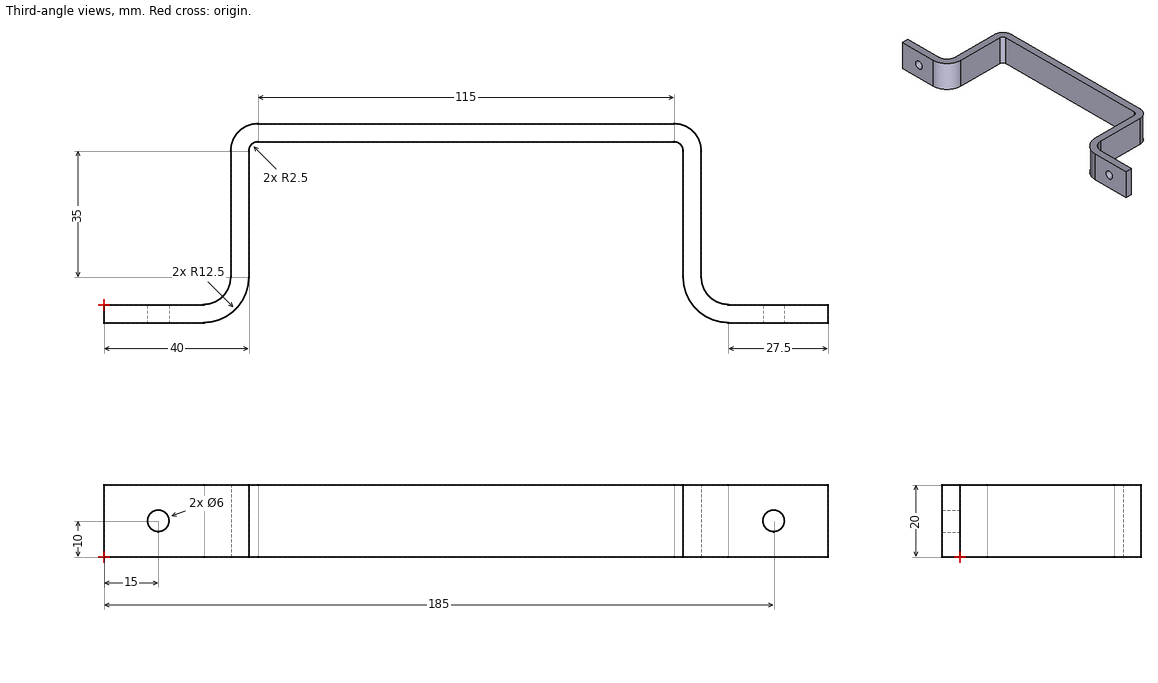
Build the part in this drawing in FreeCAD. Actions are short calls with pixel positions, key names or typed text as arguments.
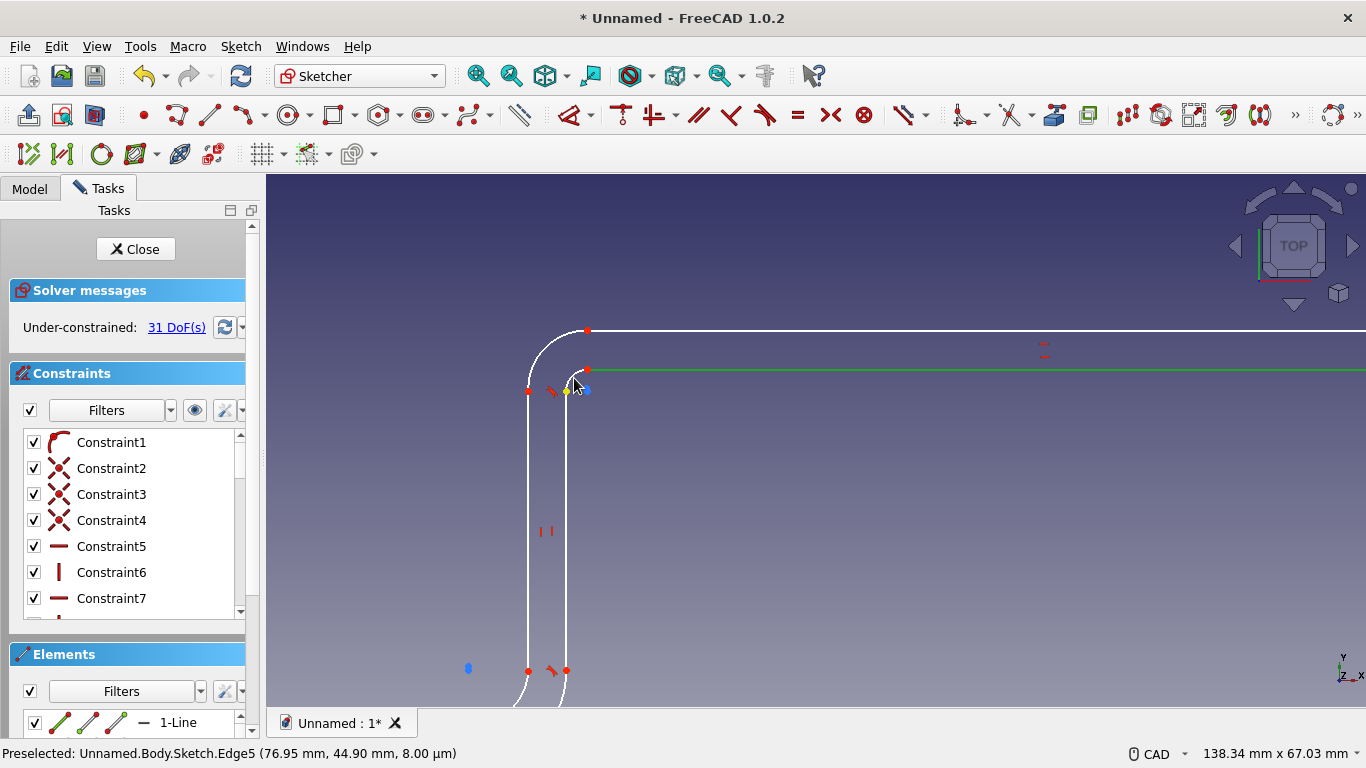
click(572, 376)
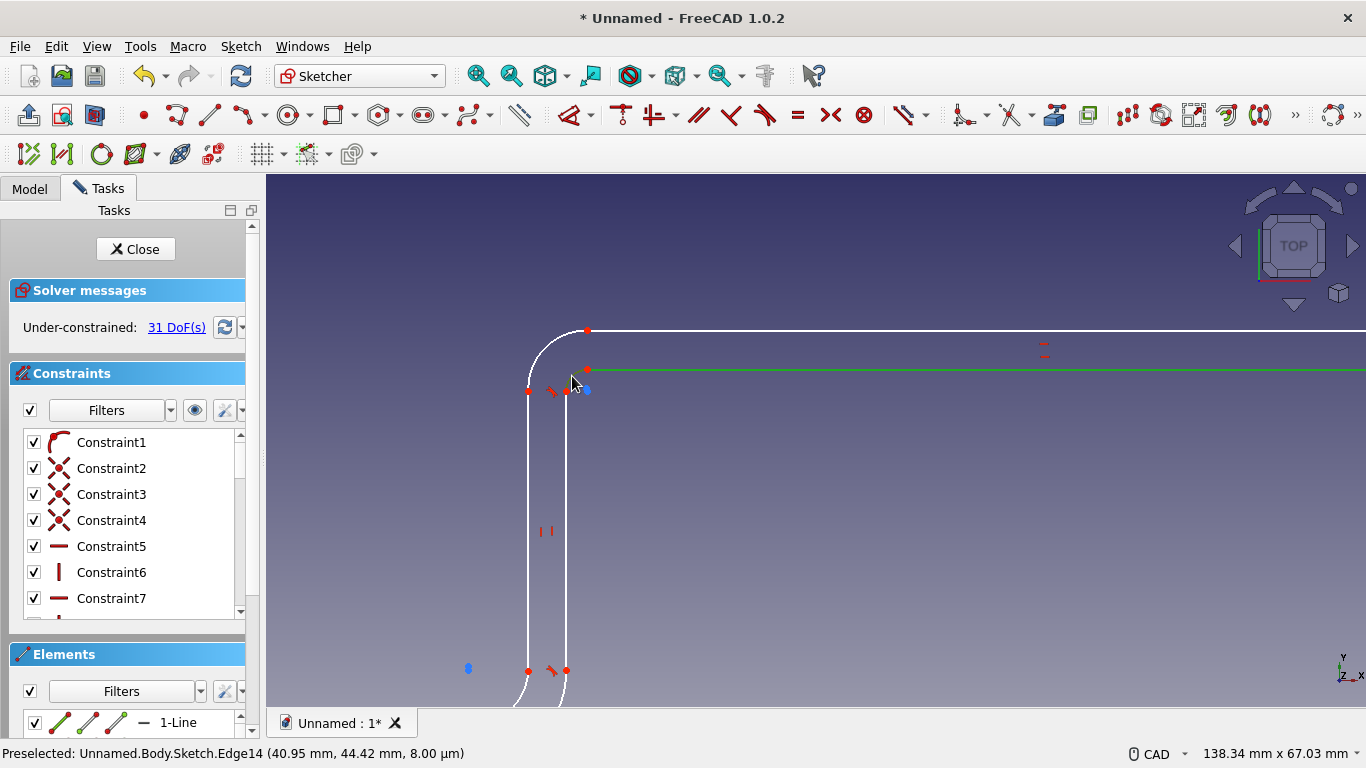
click(765, 116)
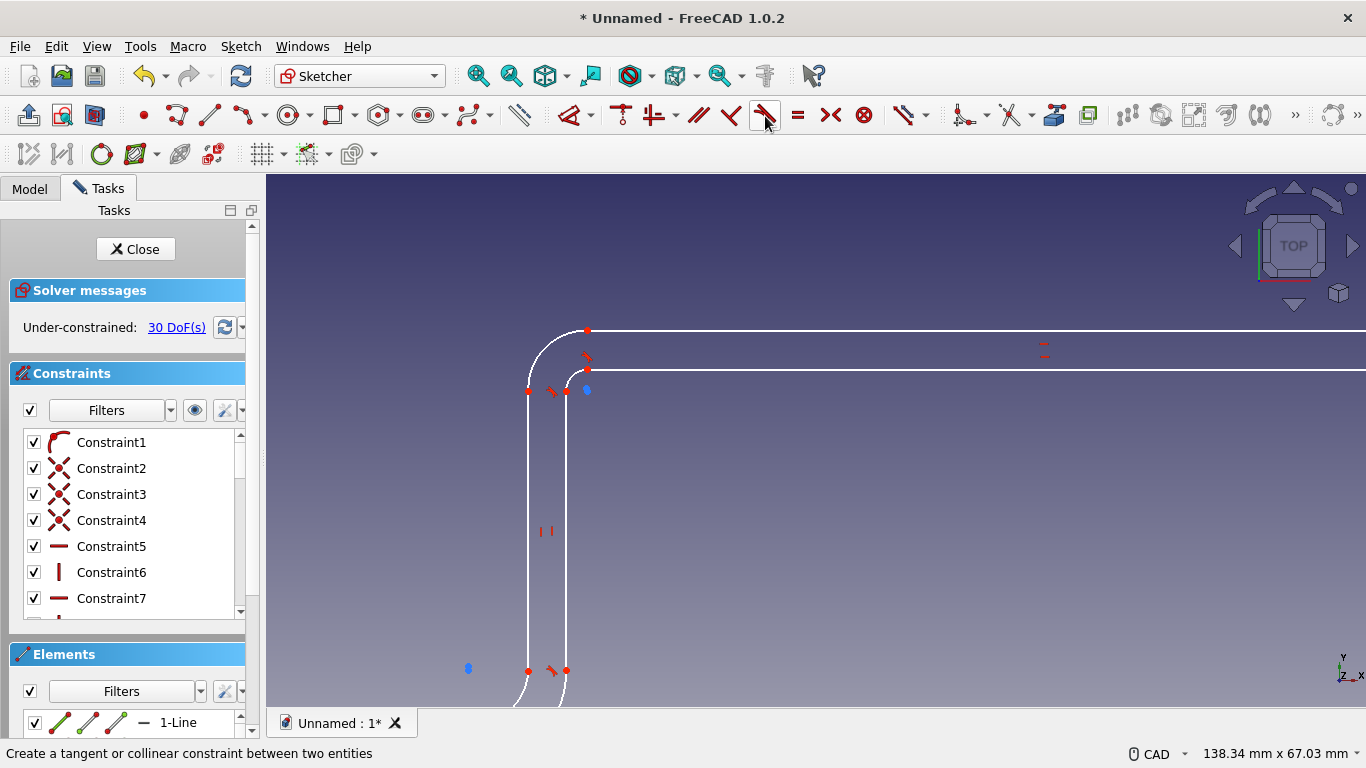
click(862, 370)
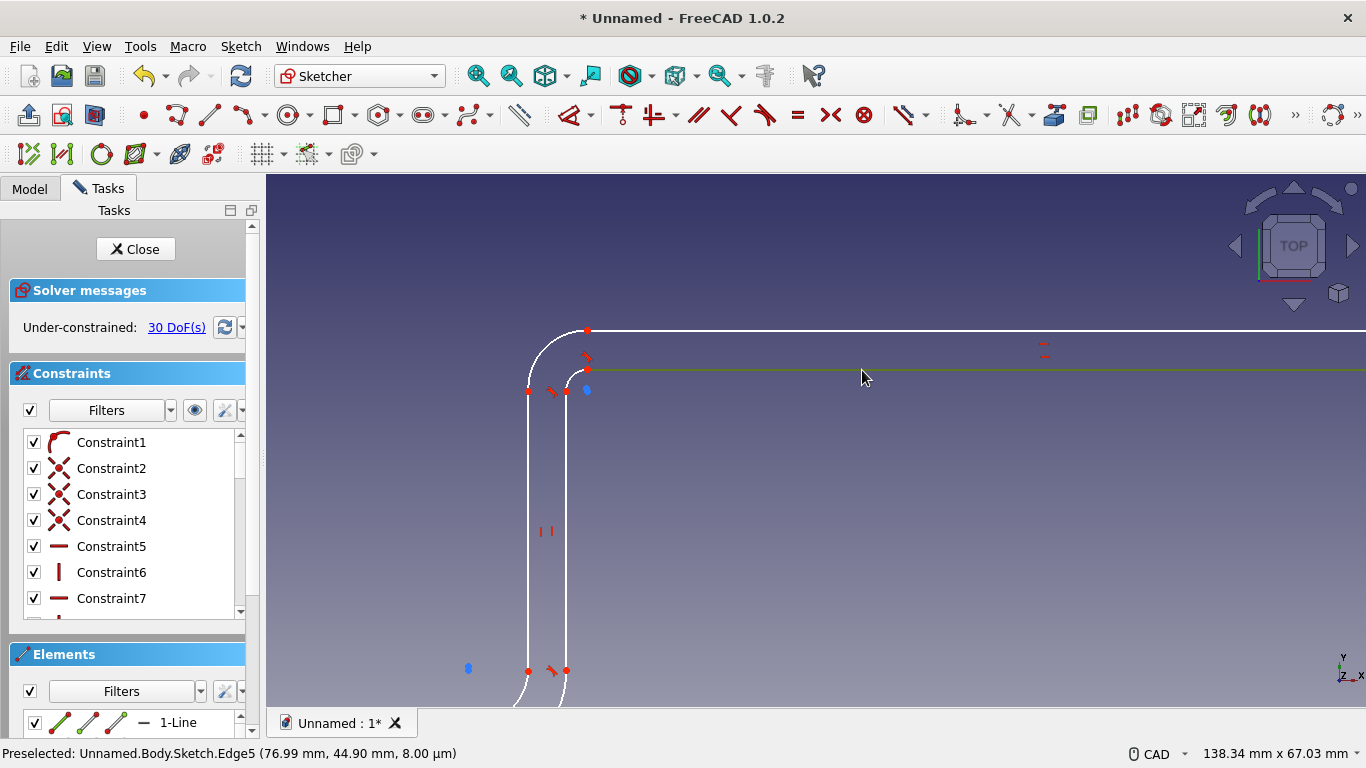
scroll(574, 378, down, 5)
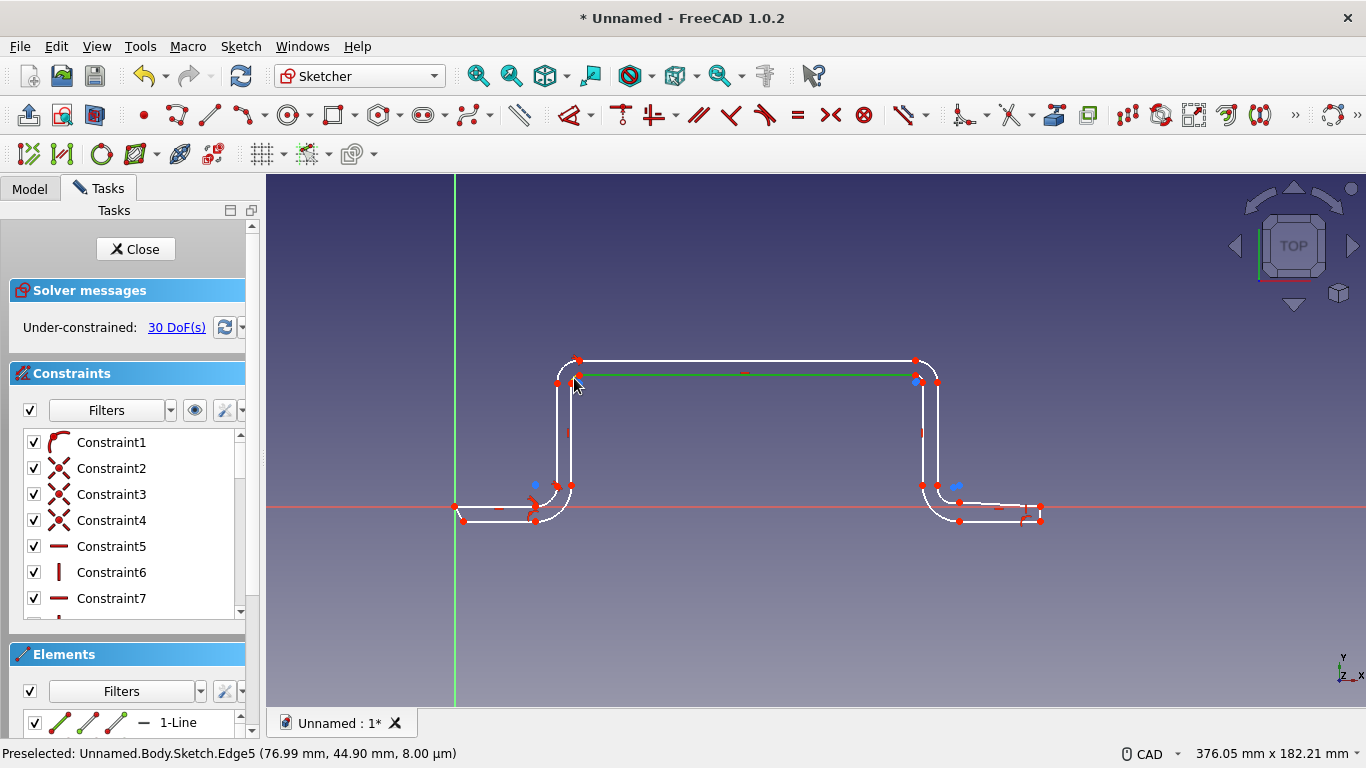
scroll(922, 379, up, 7)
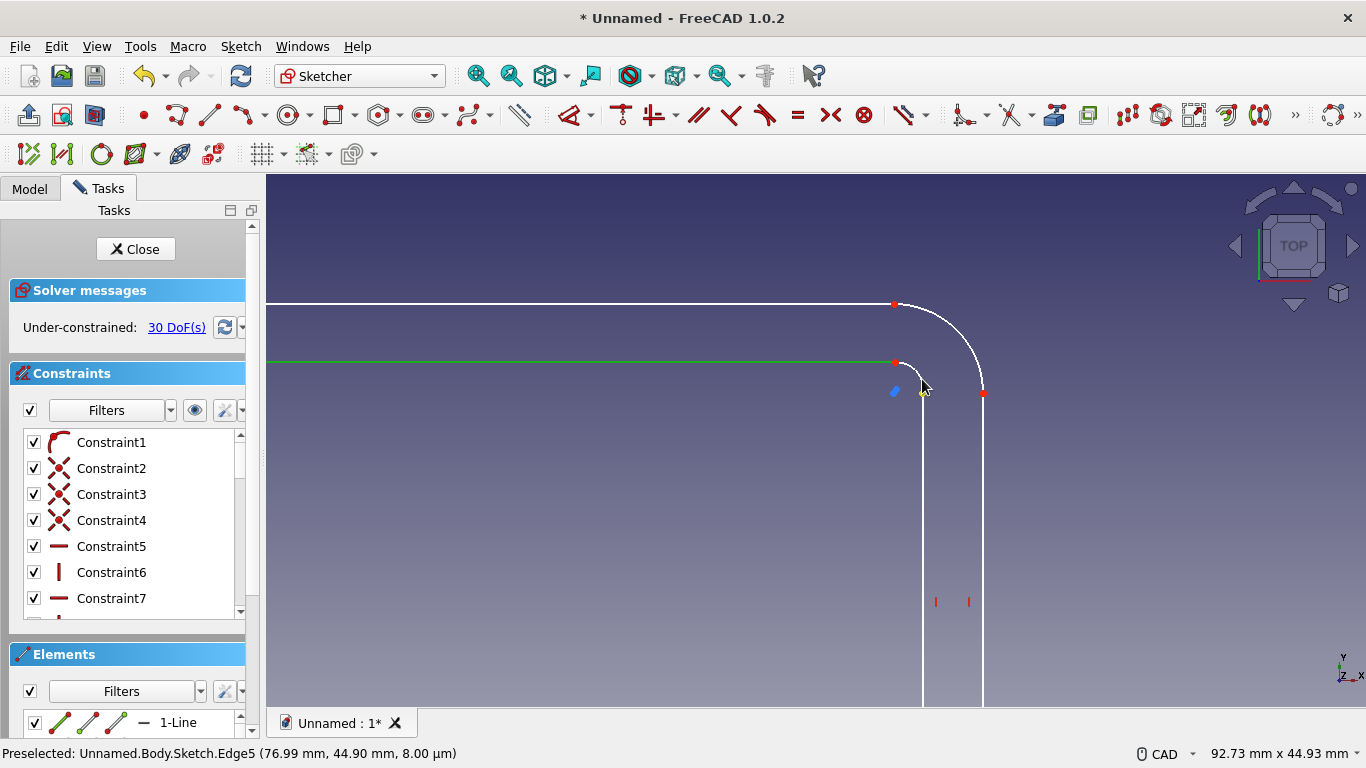
click(921, 379)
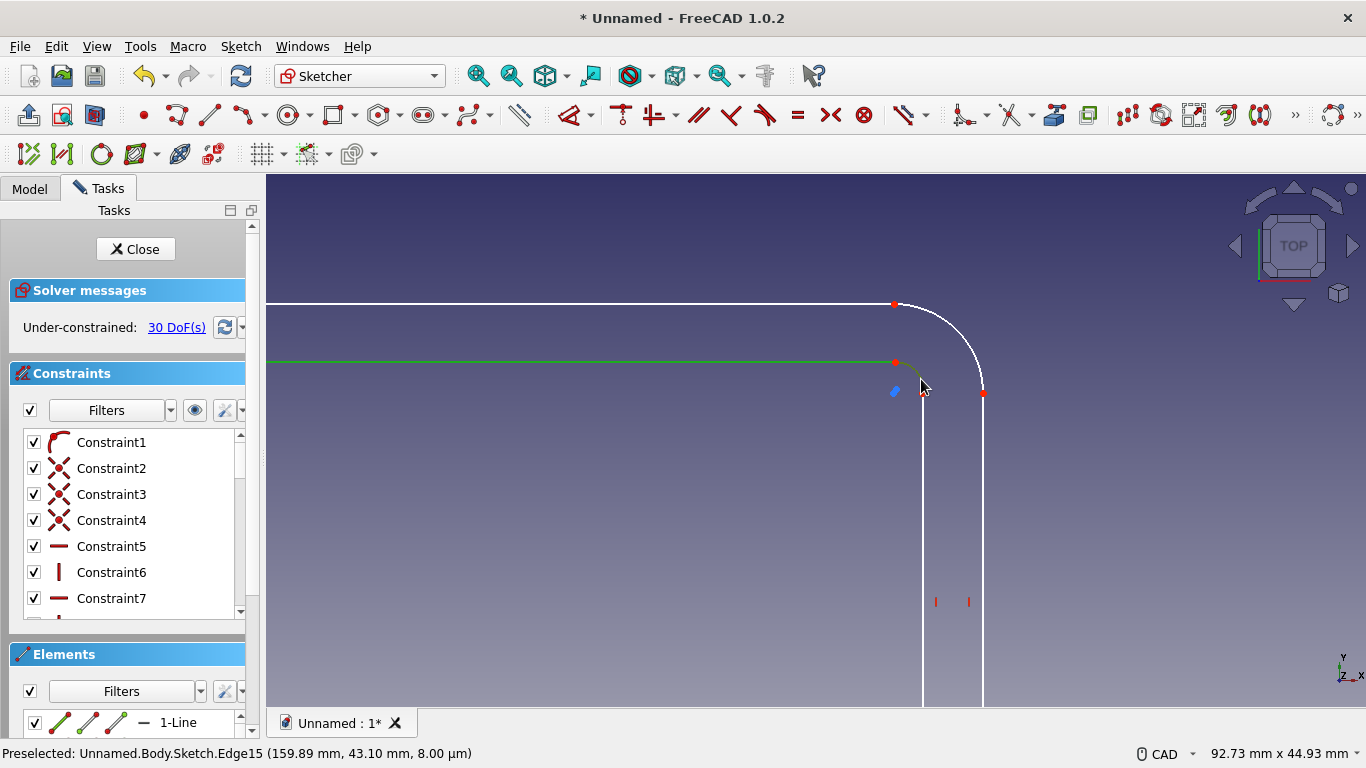
click(765, 116)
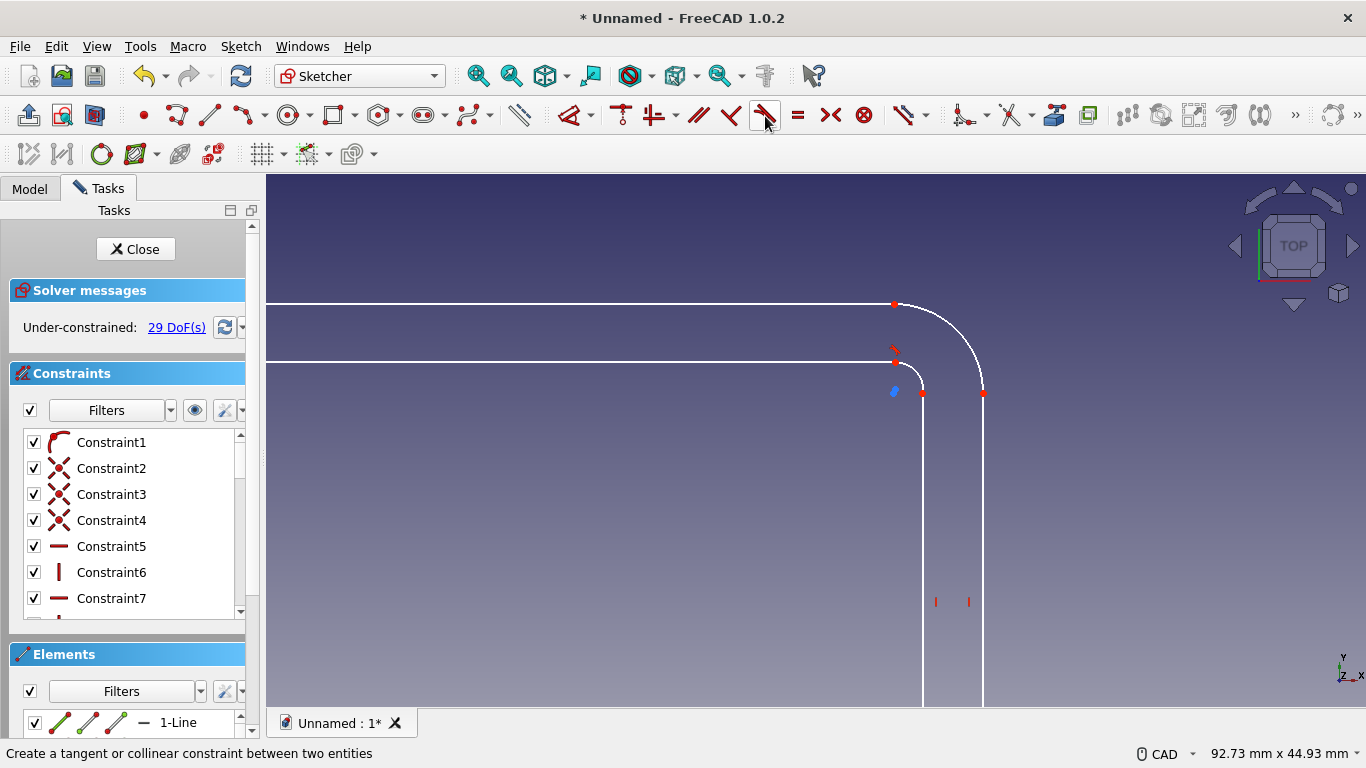
scroll(923, 379, down, 7)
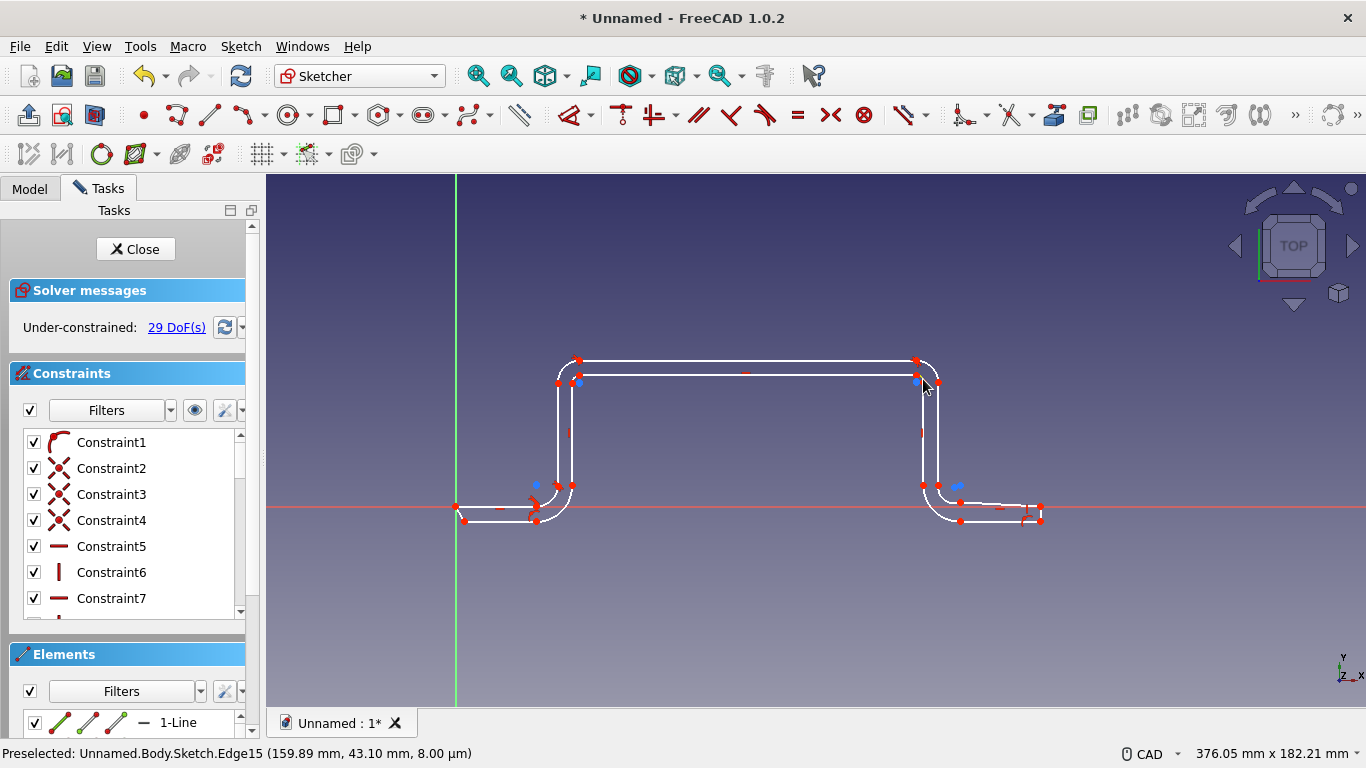
click(923, 414)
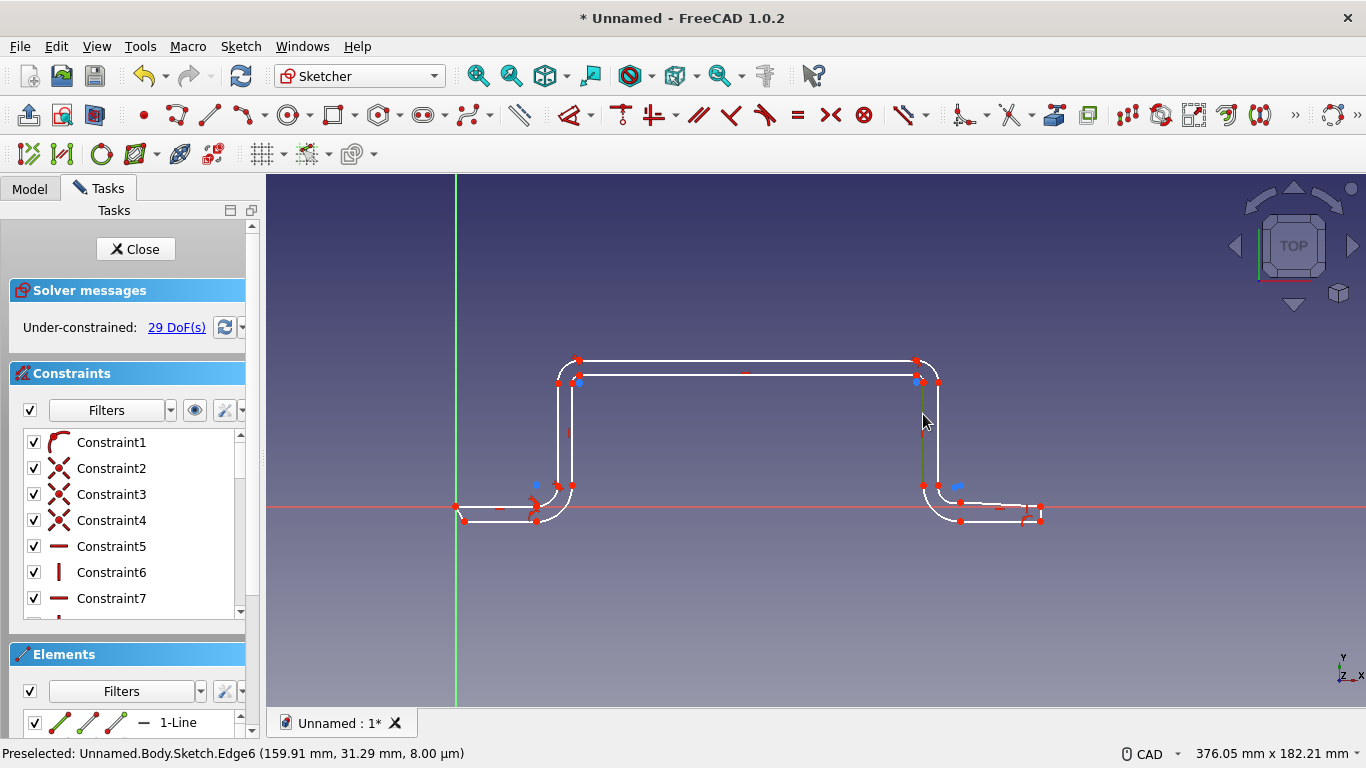
scroll(922, 377, up, 5)